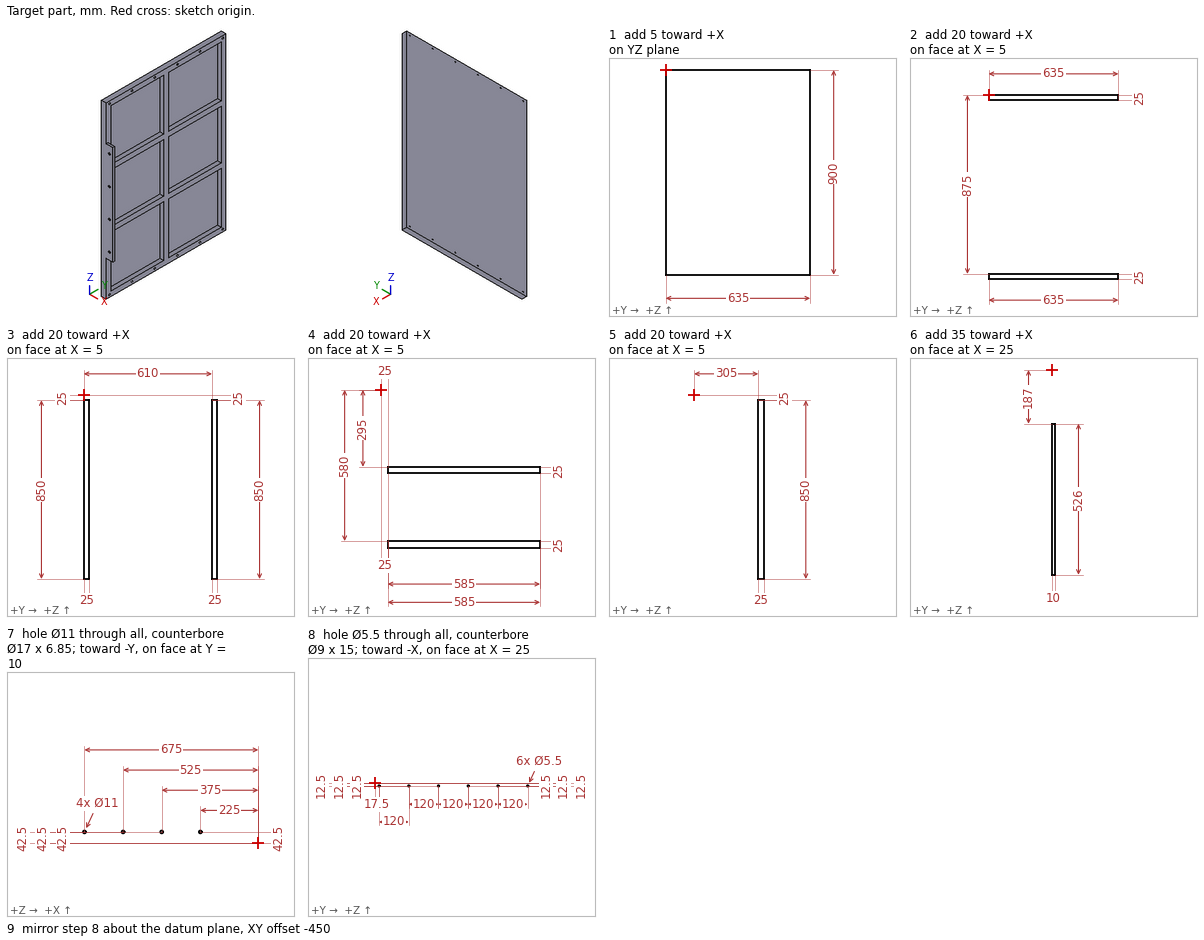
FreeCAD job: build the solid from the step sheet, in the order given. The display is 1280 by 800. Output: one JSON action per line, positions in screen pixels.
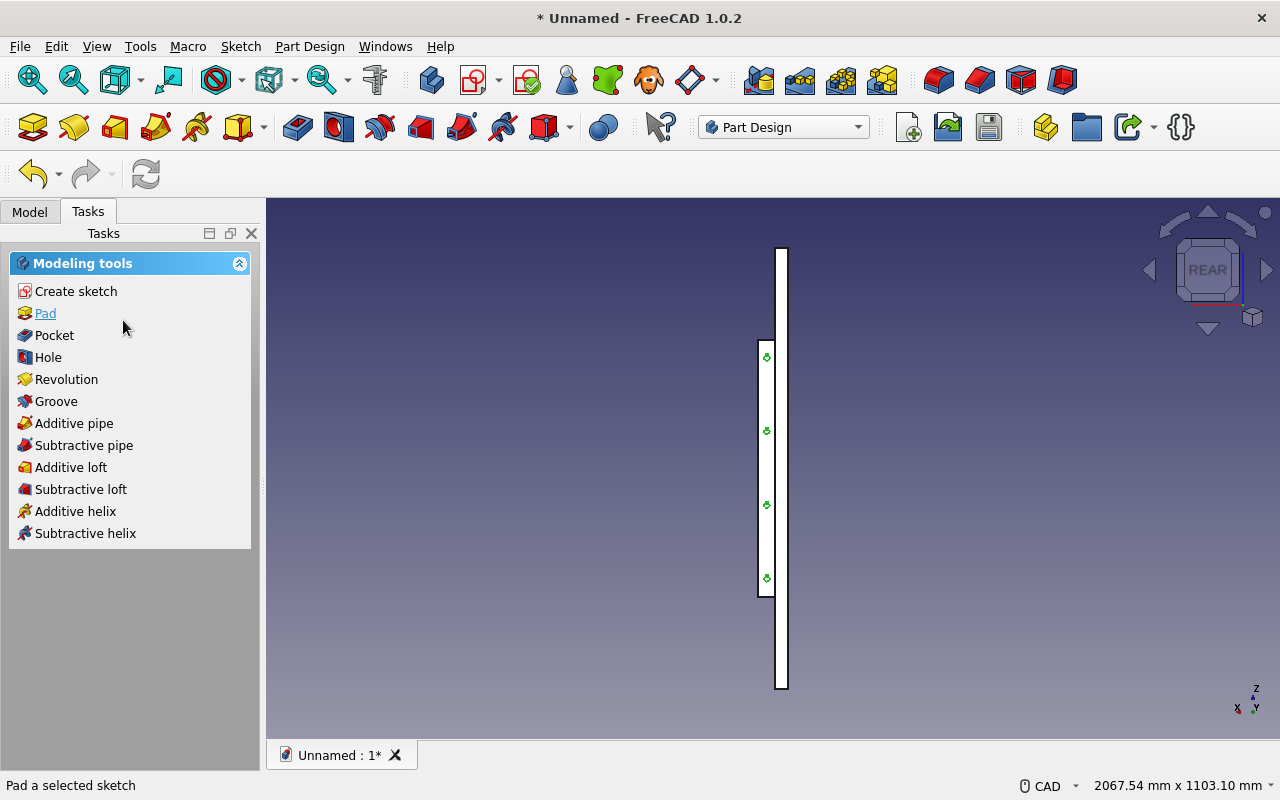
{"action": "left_click", "coordinate": [339, 128]}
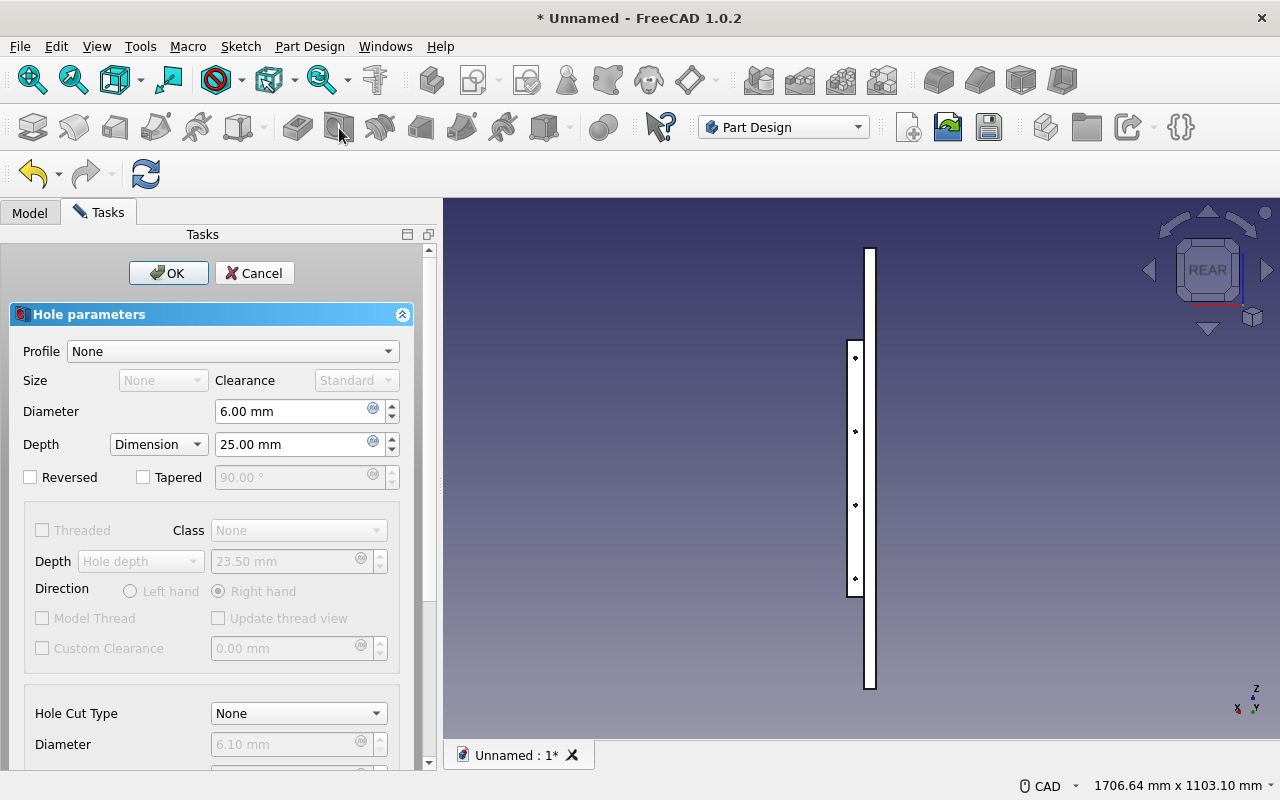
{"action": "triple_click", "coordinate": [300, 412]}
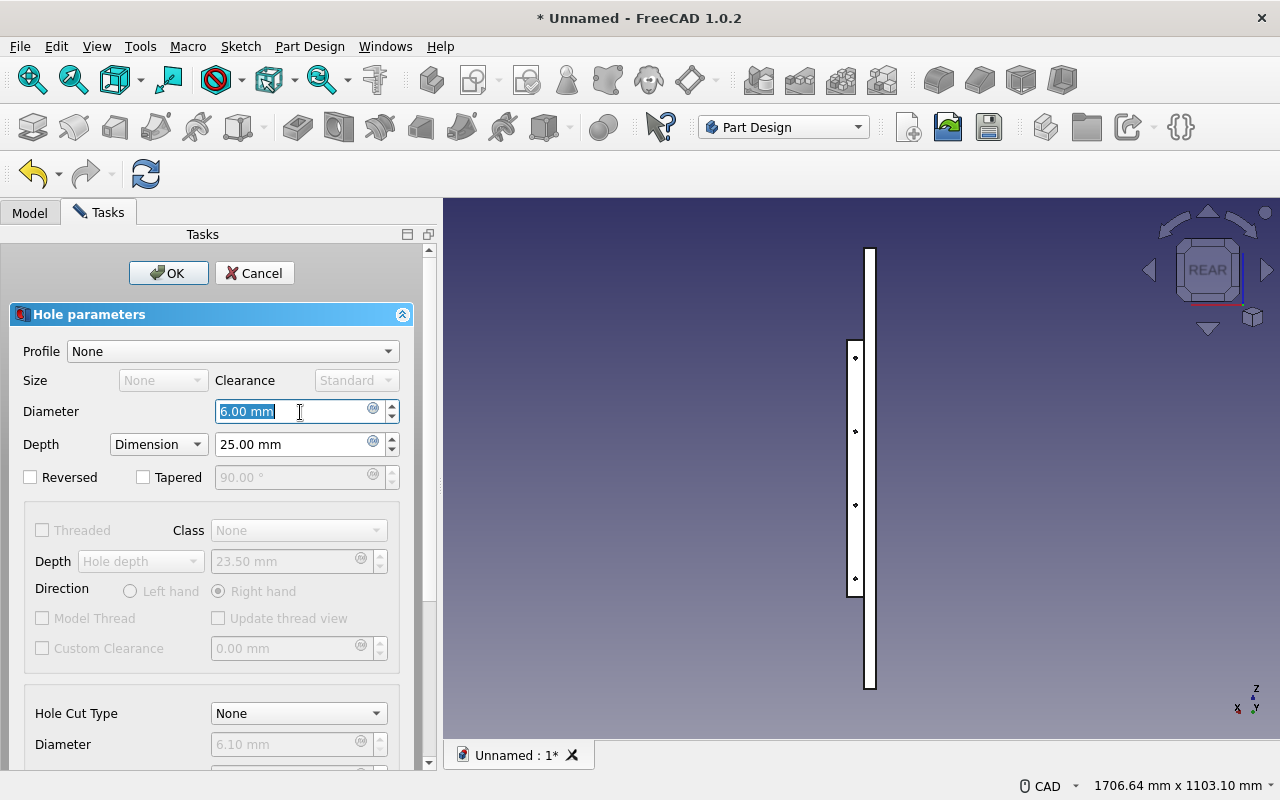
{"action": "type", "text": "11"}
{"action": "key", "text": "Tab"}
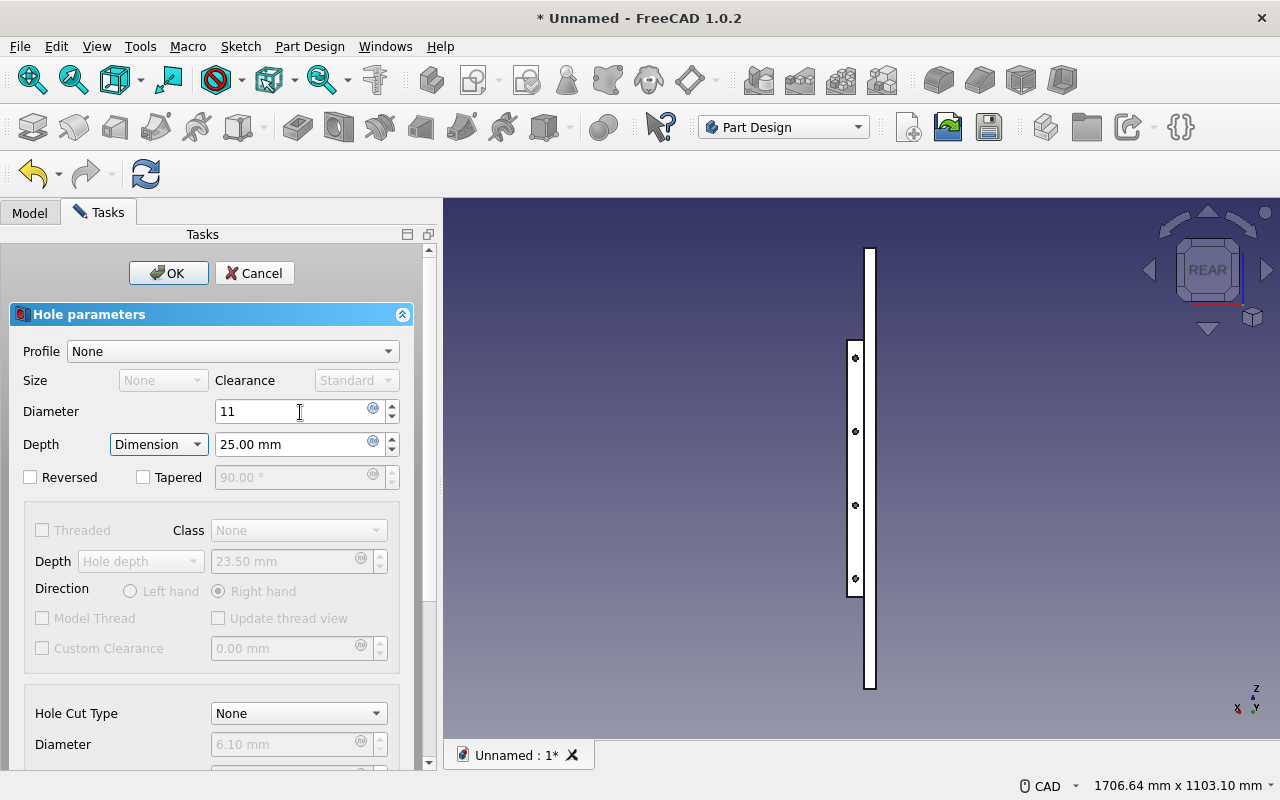
{"action": "left_click", "coordinate": [160, 444]}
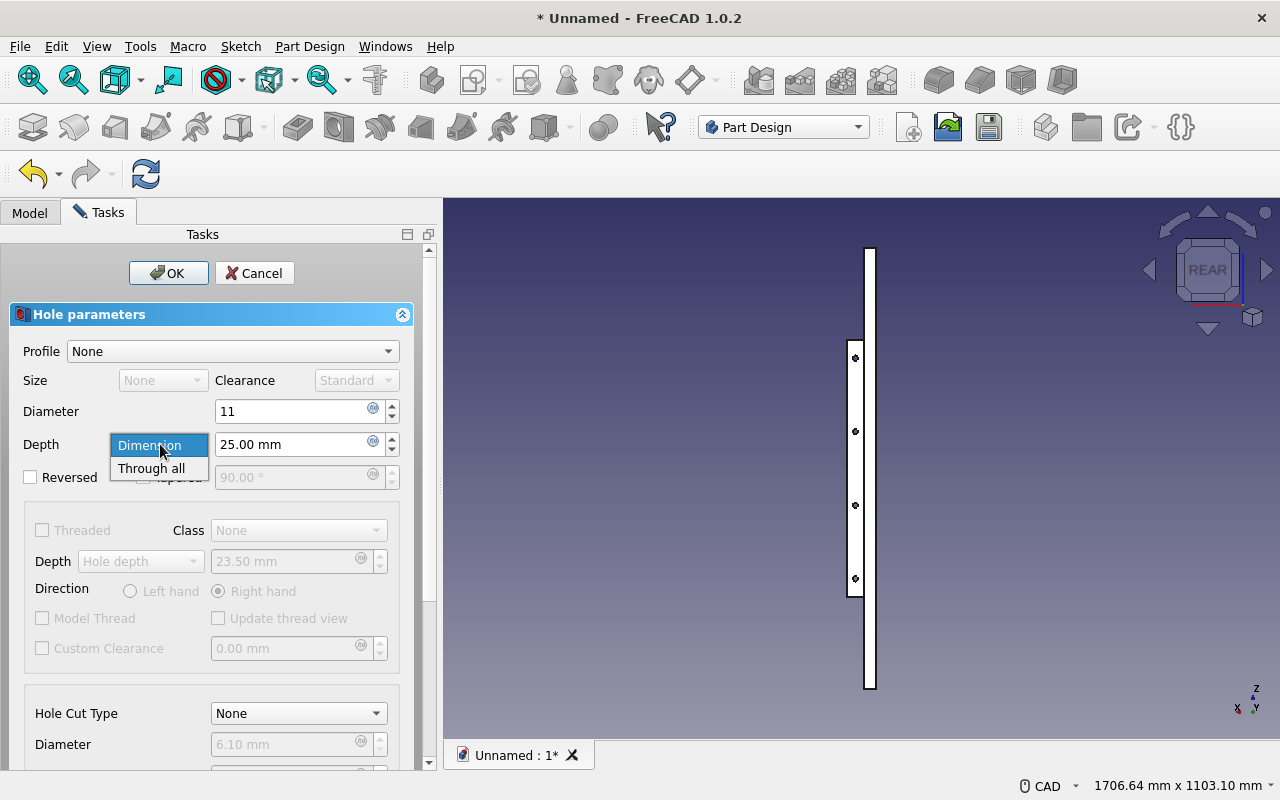
{"action": "left_click", "coordinate": [158, 468]}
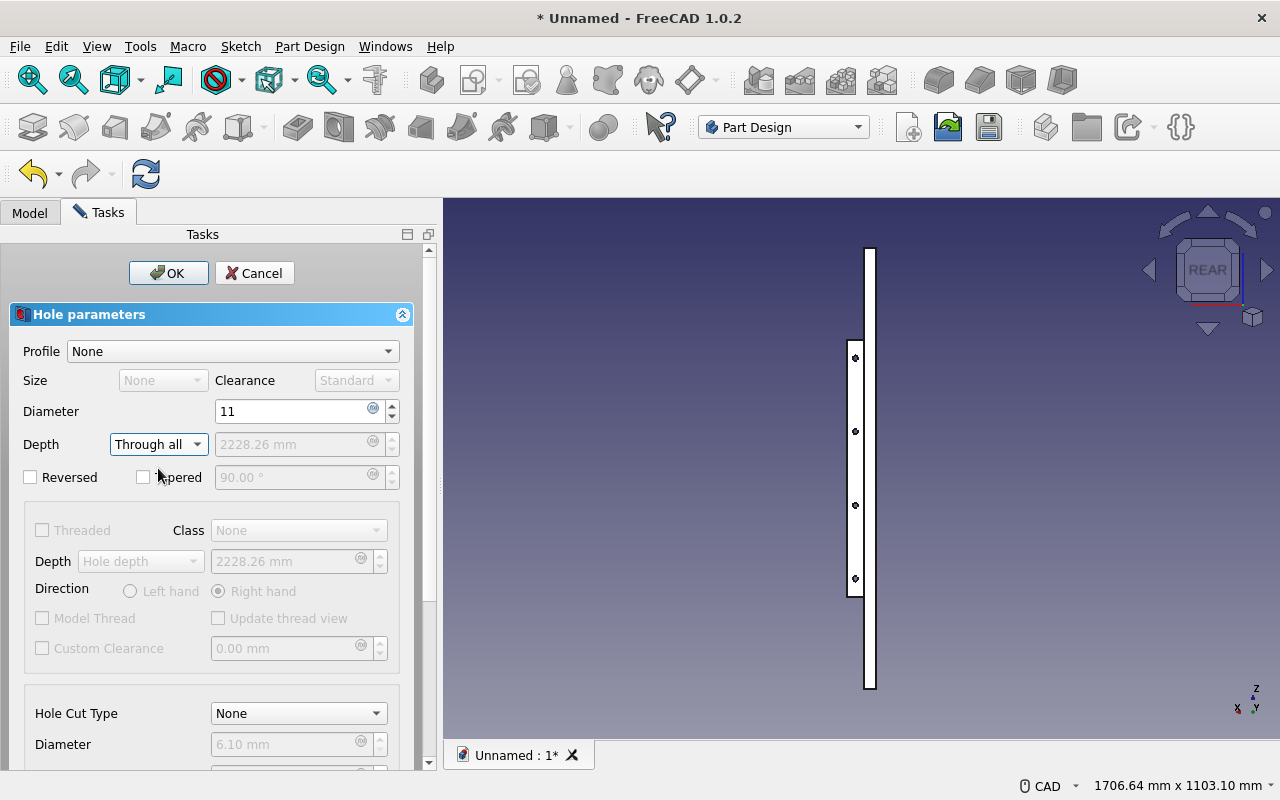
{"action": "left_click", "coordinate": [300, 714]}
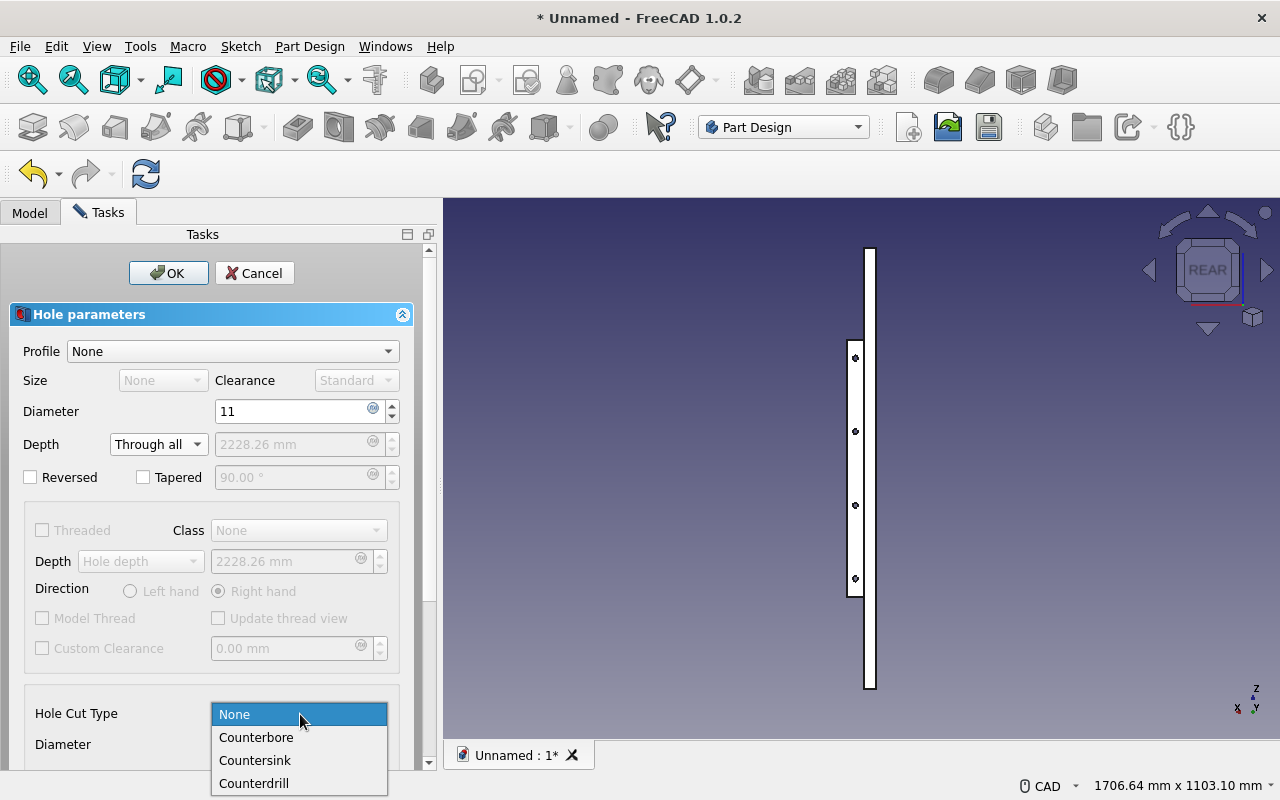
{"action": "left_click", "coordinate": [298, 738]}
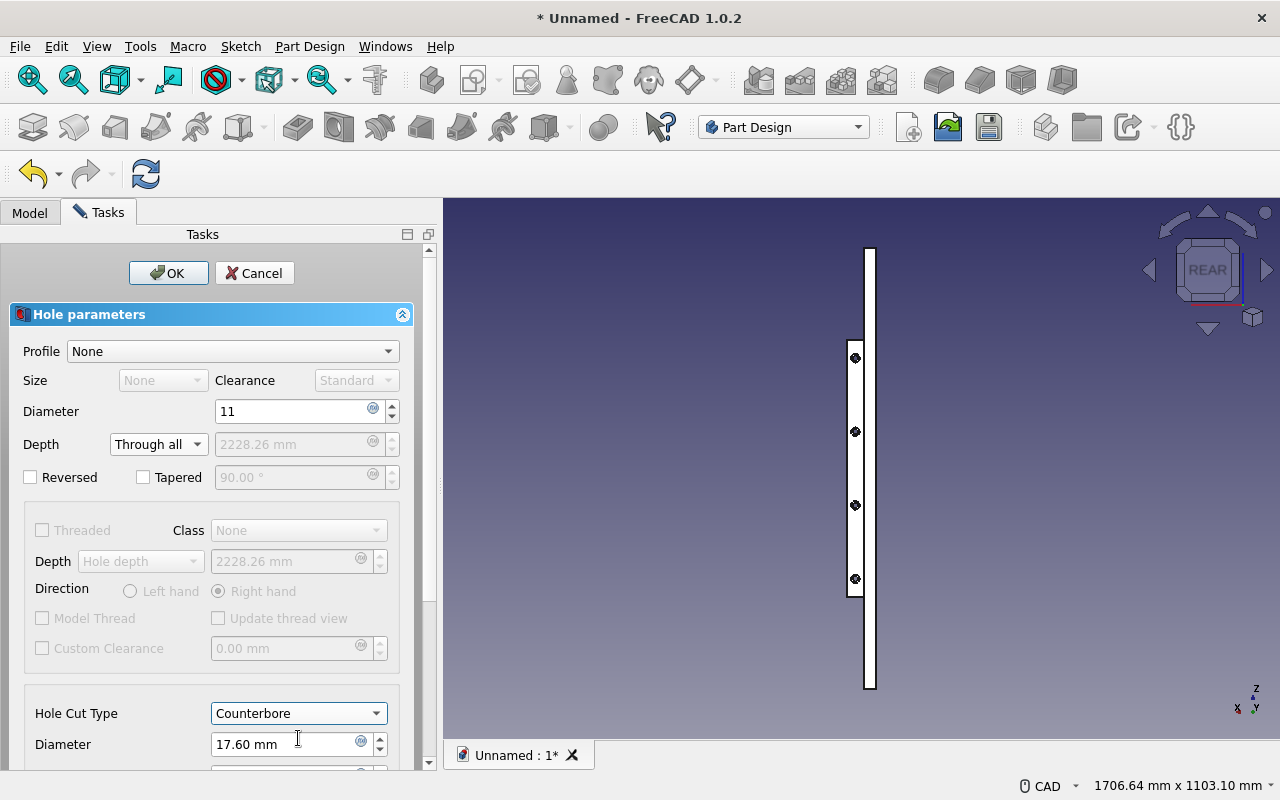
{"action": "triple_click", "coordinate": [292, 744]}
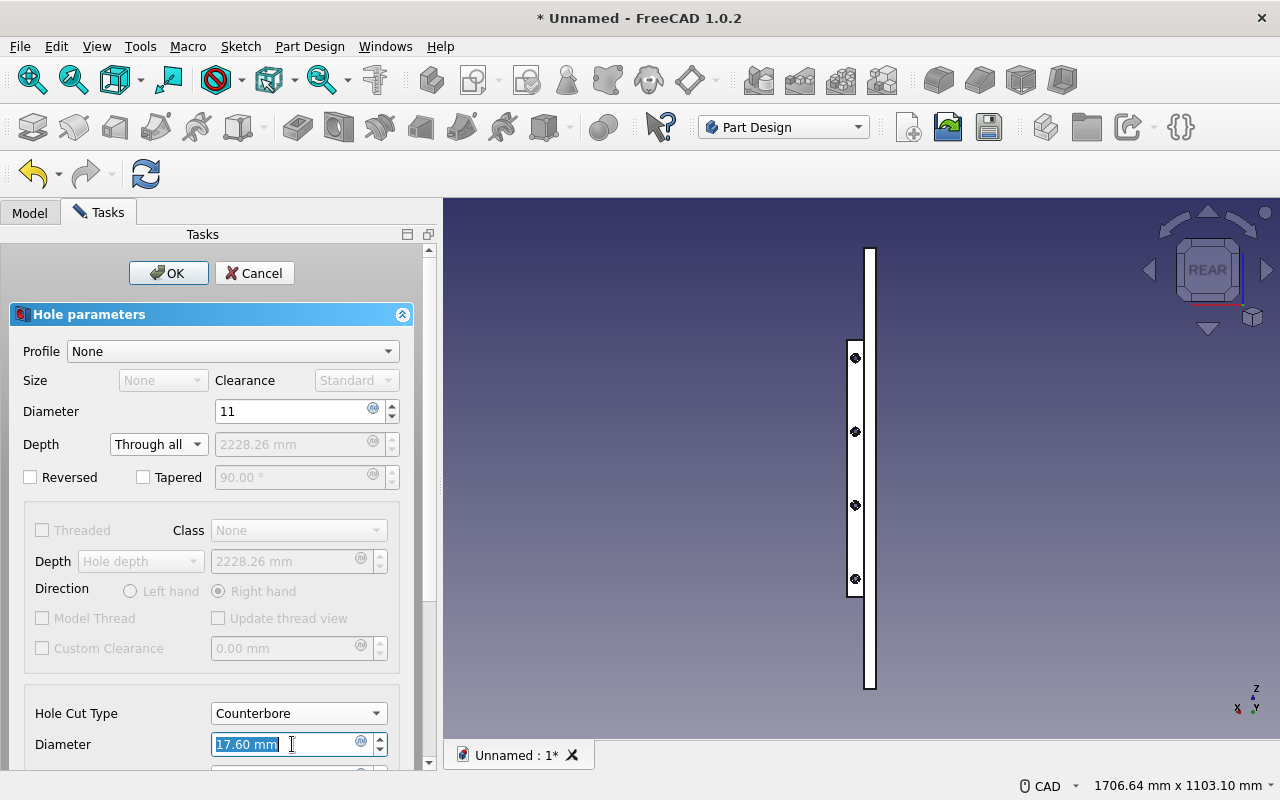
{"action": "type", "text": "17"}
{"action": "key", "text": "Tab"}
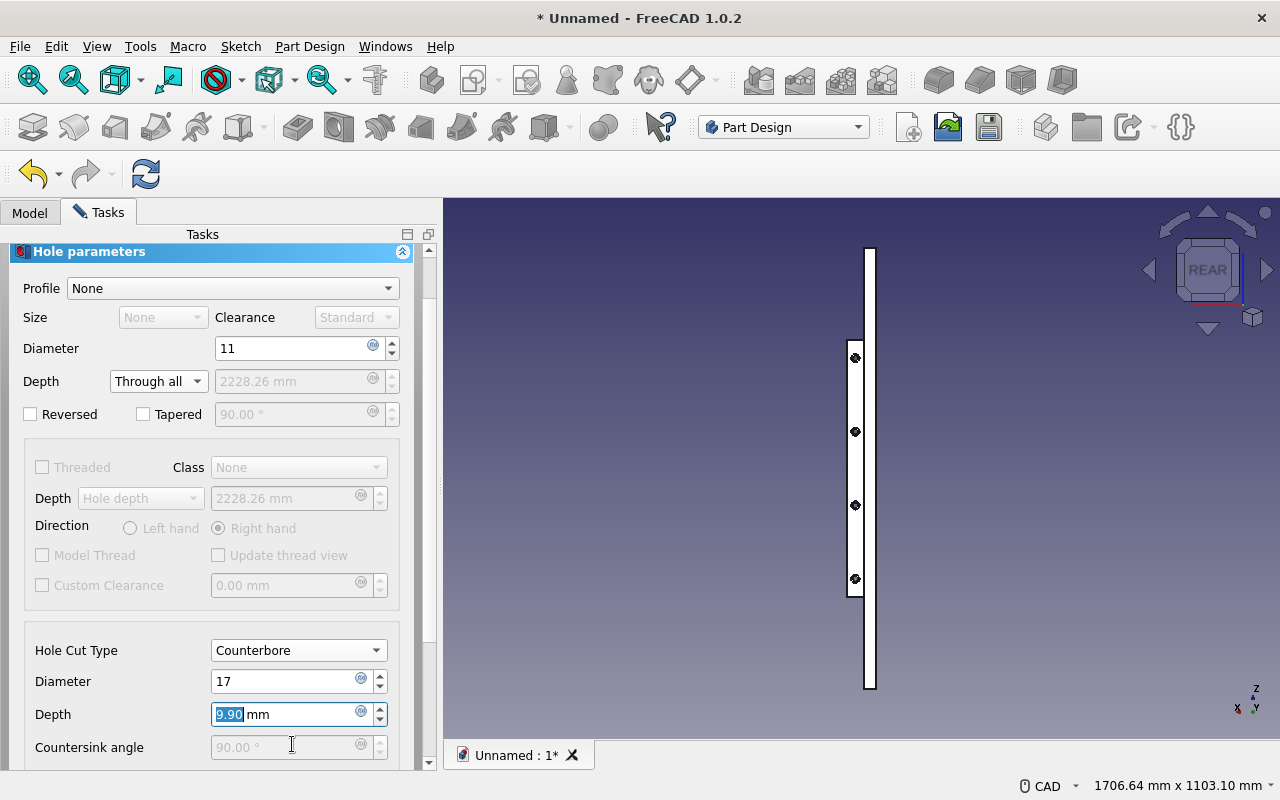
{"action": "type", "text": "6.85"}
{"action": "key", "text": "Tab"}